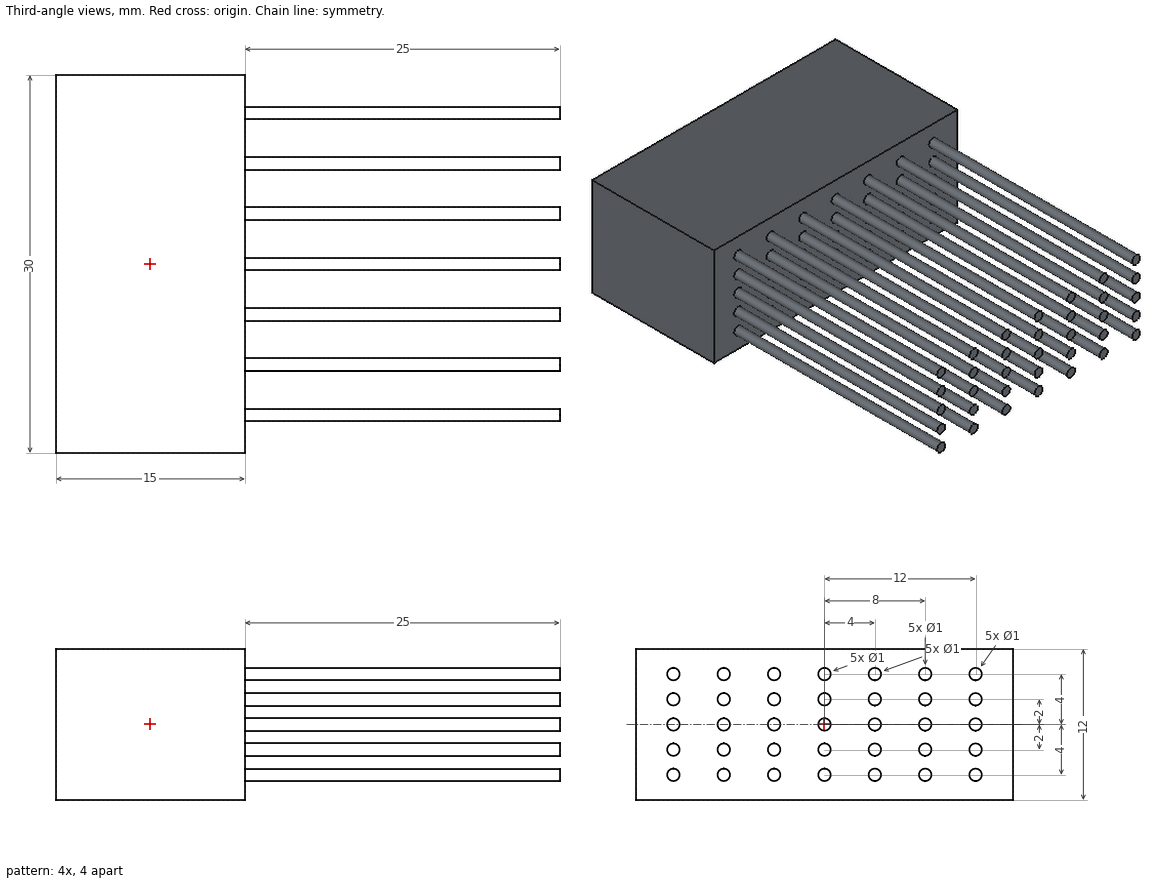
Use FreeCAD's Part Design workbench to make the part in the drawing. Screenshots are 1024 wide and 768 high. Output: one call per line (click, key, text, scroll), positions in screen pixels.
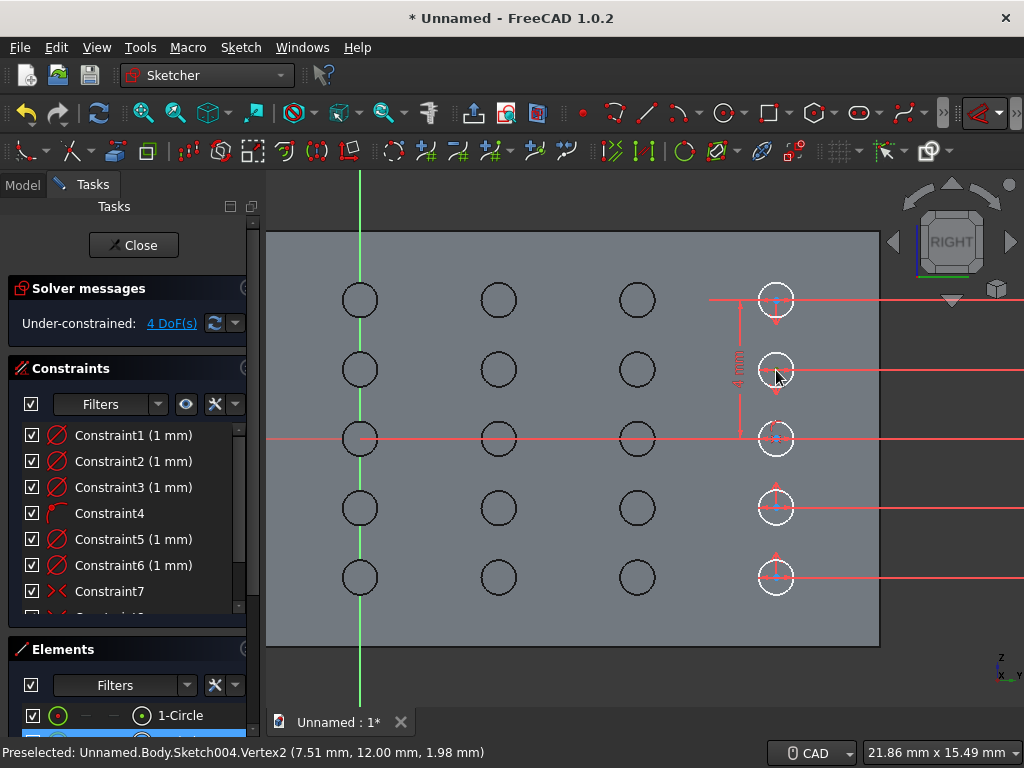
key(i)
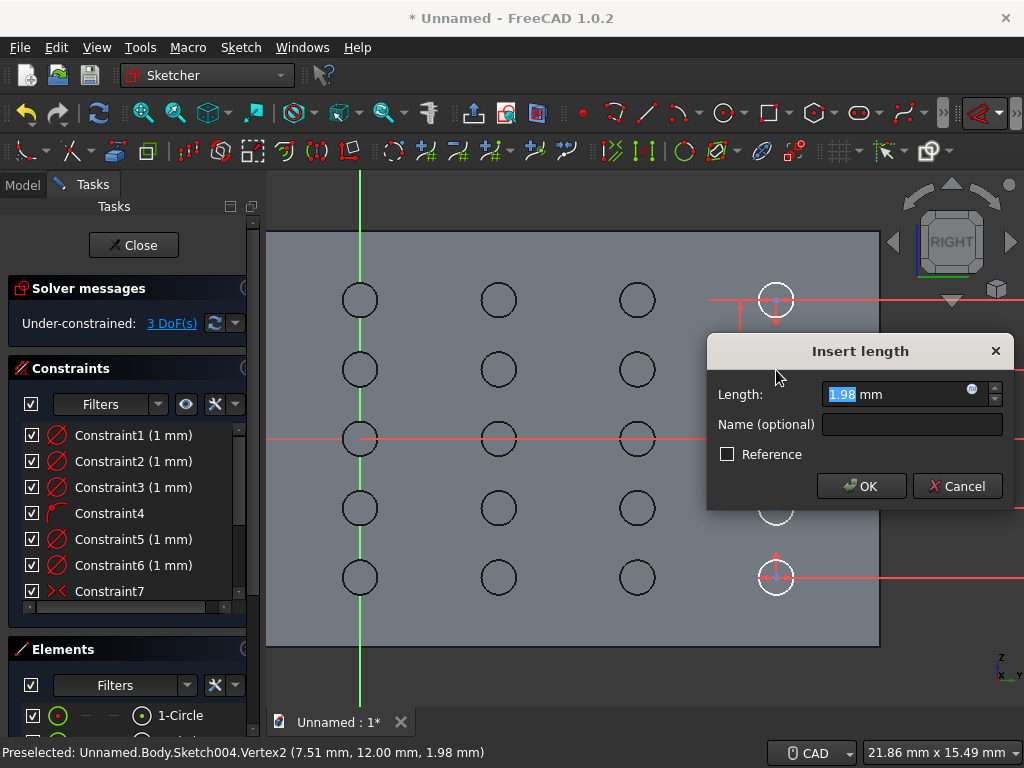
text(2)
key(Return)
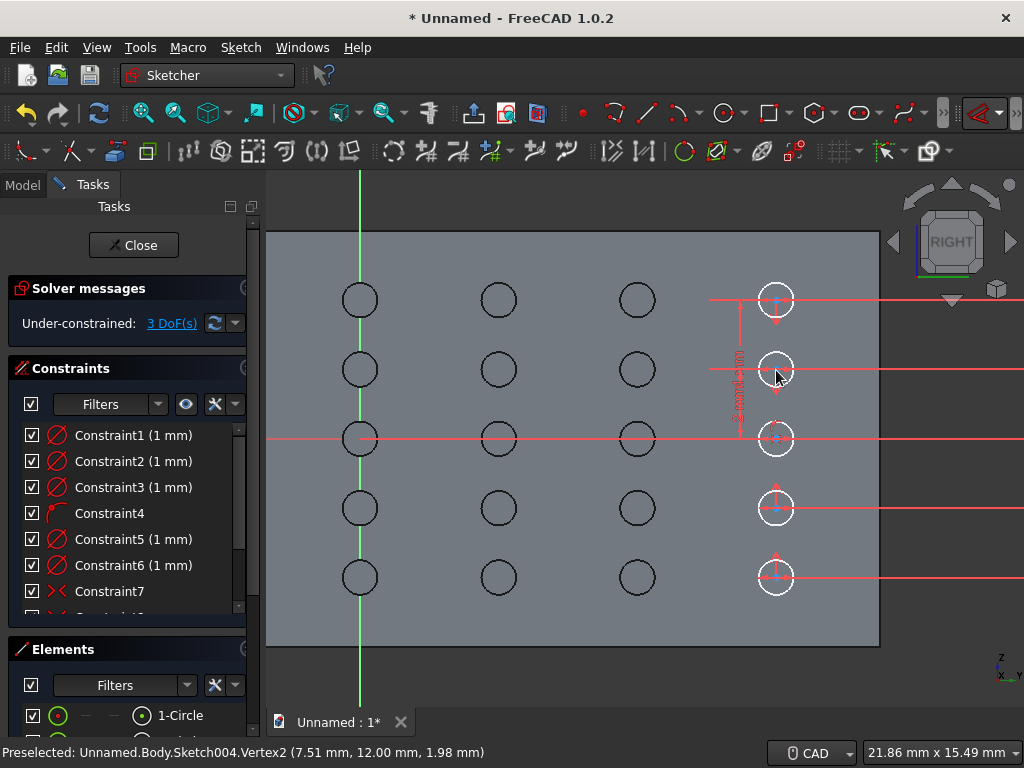
click(776, 300)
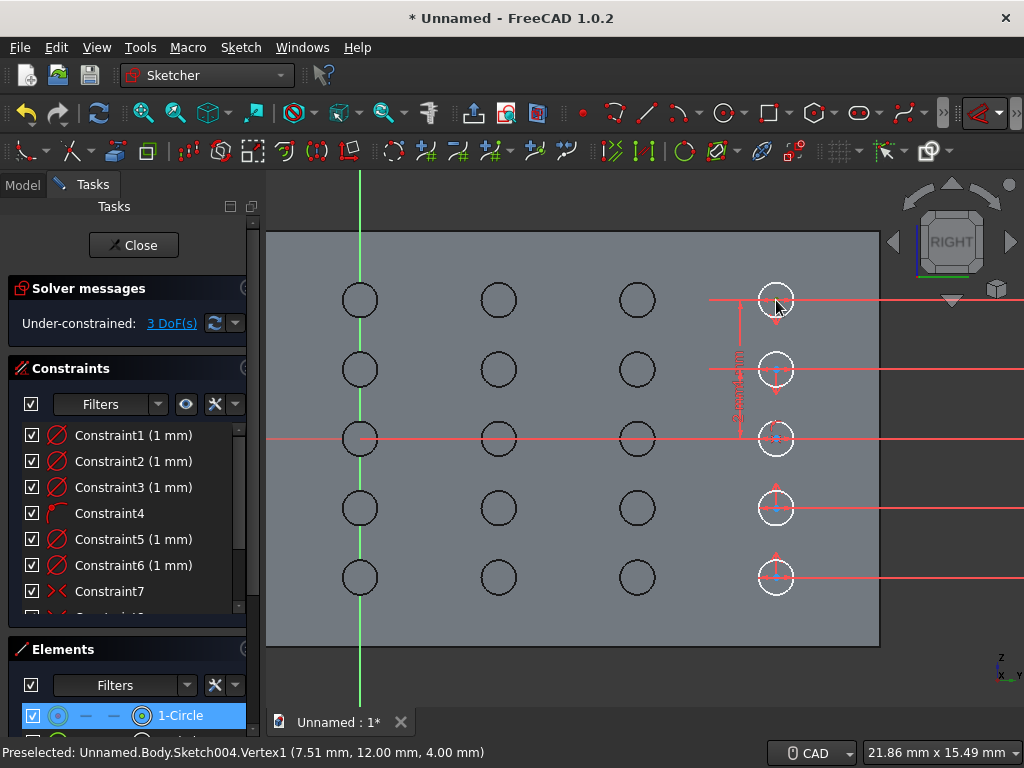
click(1002, 114)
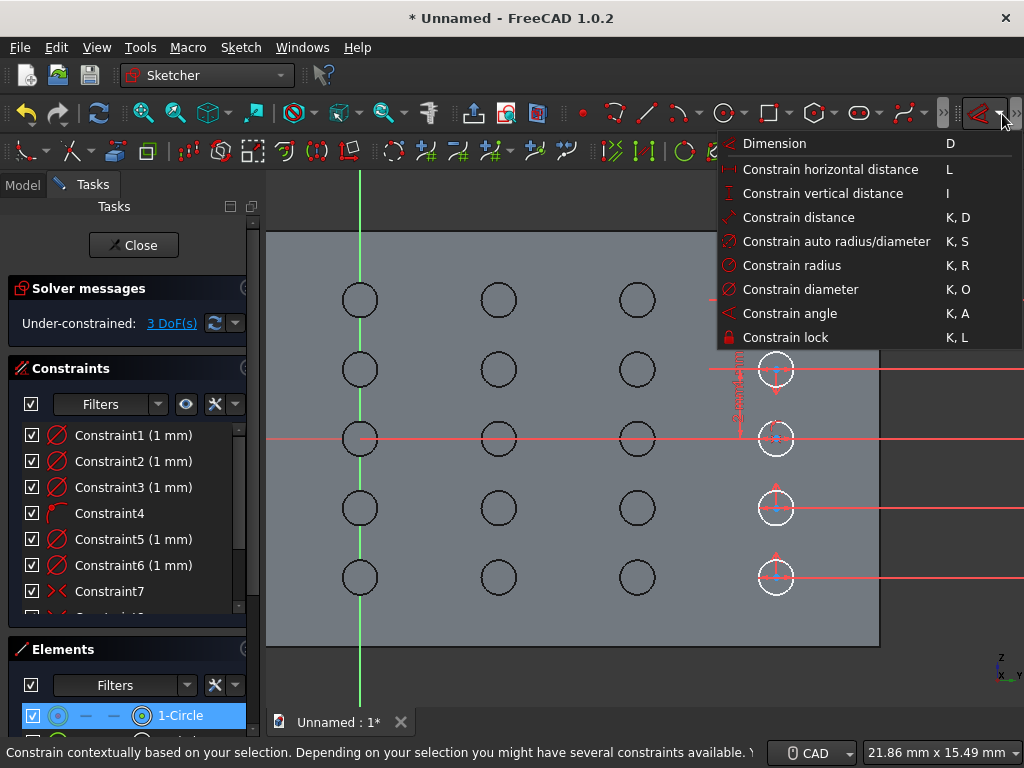
click(870, 169)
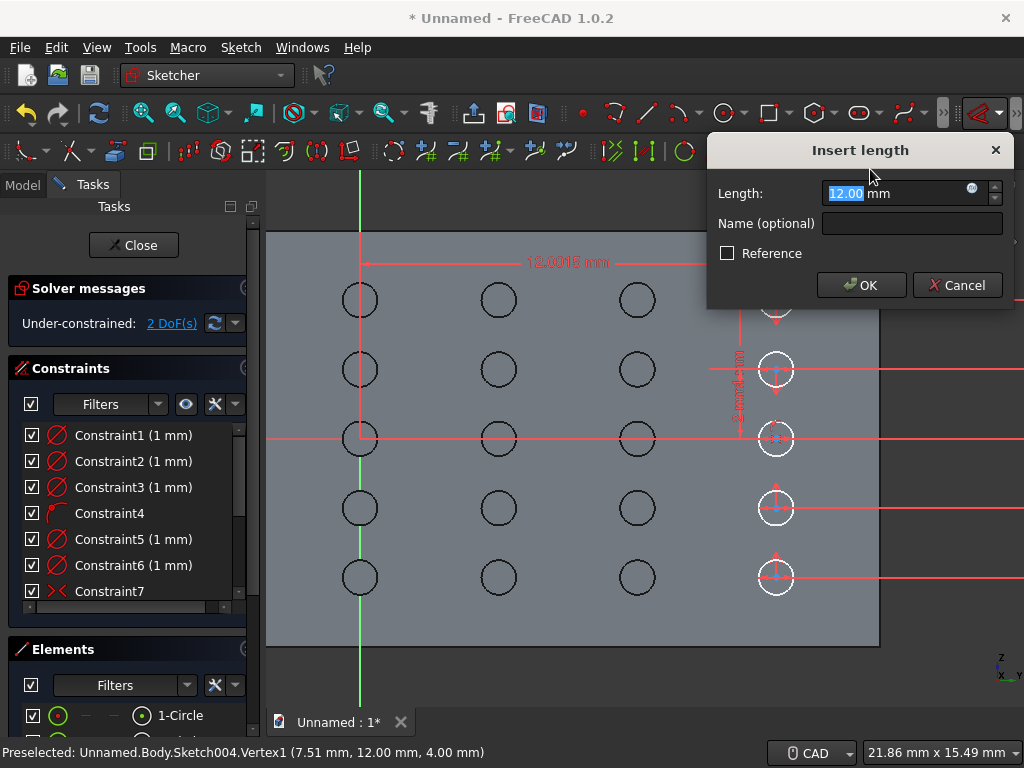
text(12)
key(Return)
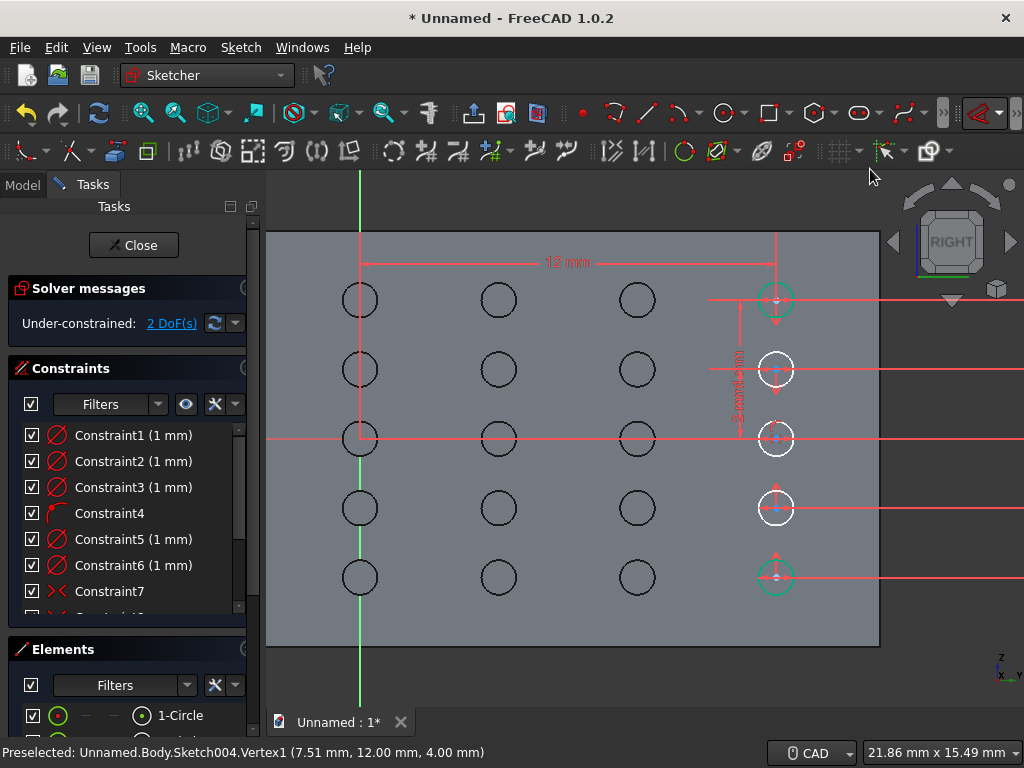
click(776, 369)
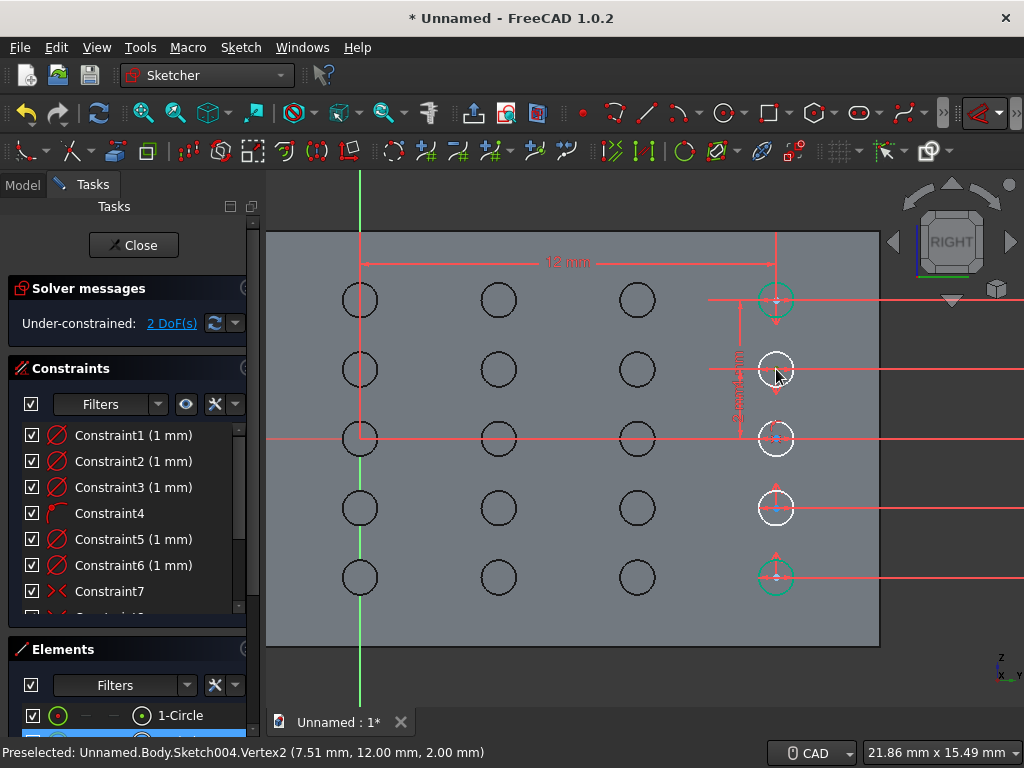
key(l)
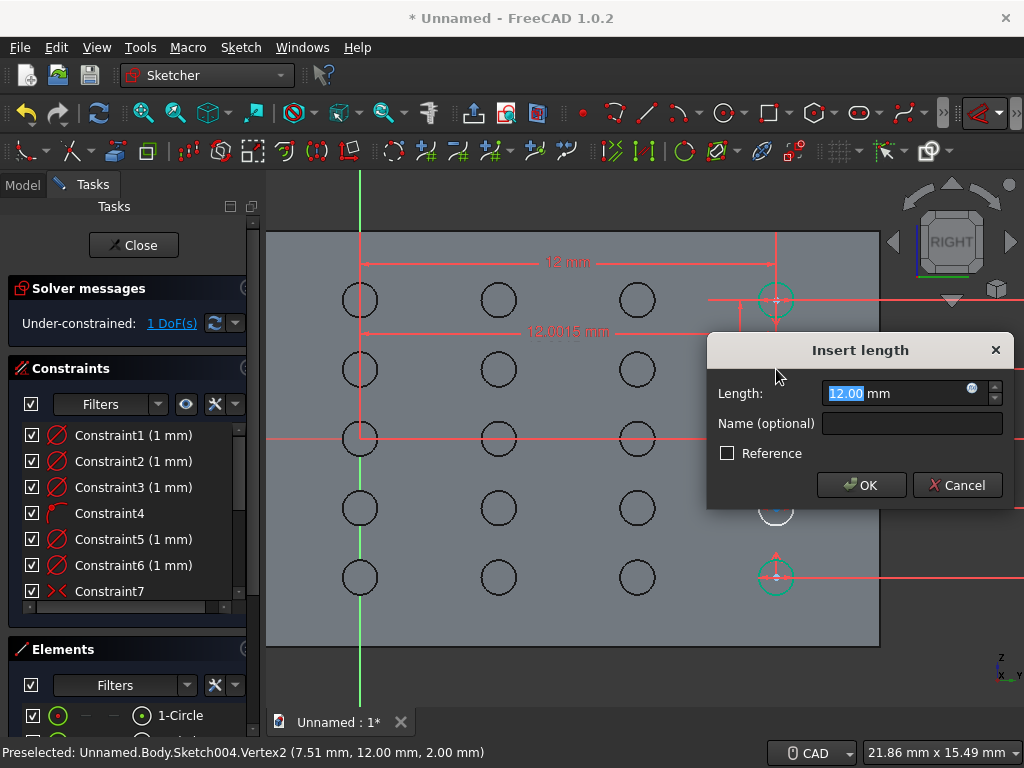
text(12)
key(Return)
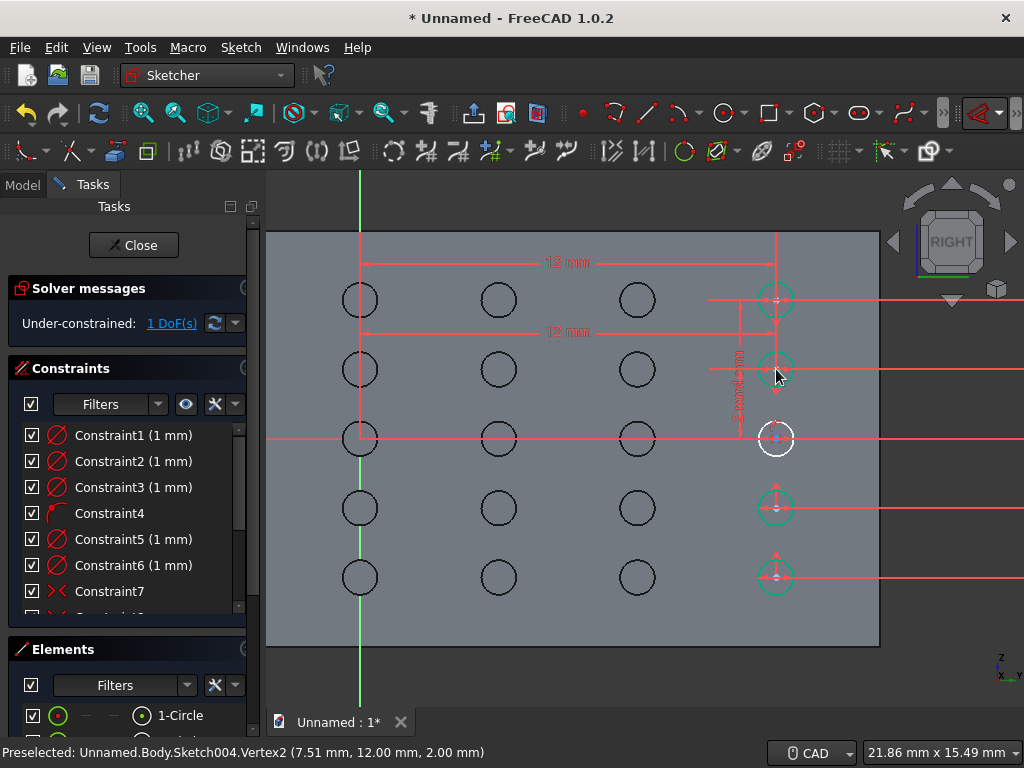
click(776, 439)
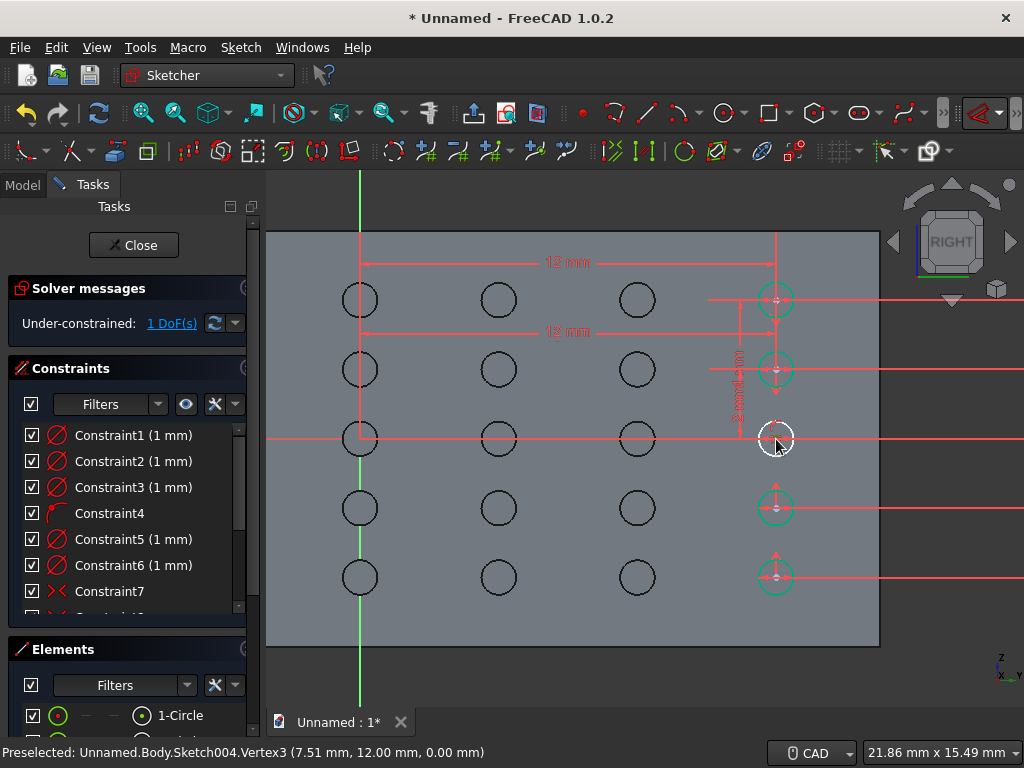
key(l)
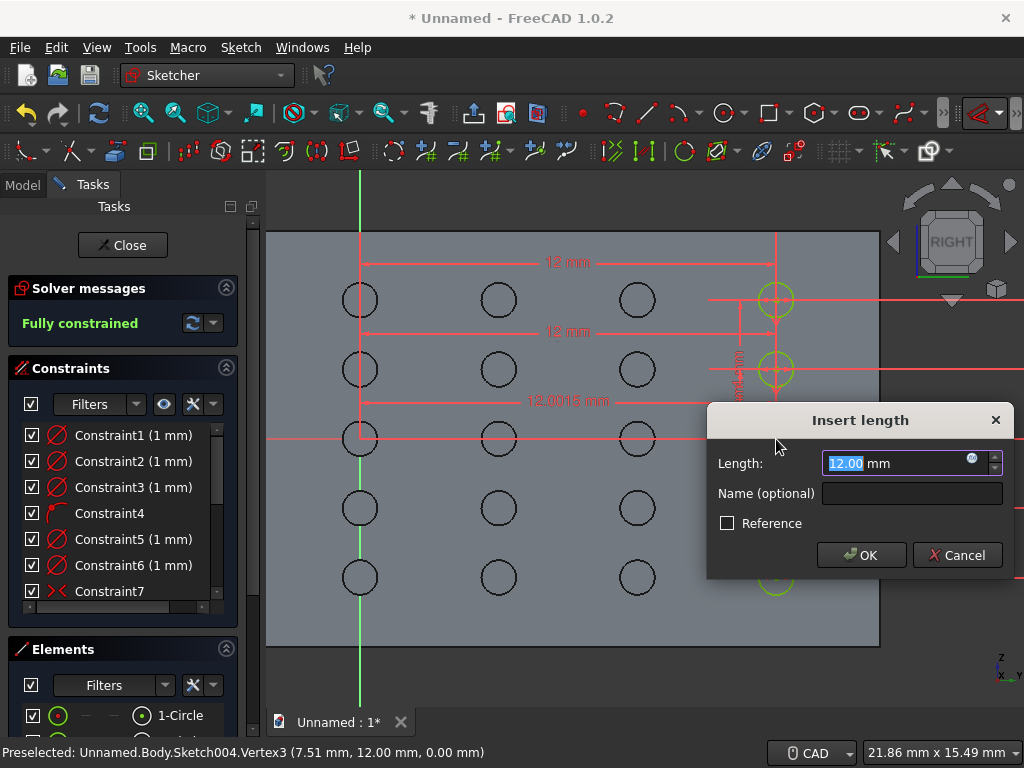
text(12)
key(Return)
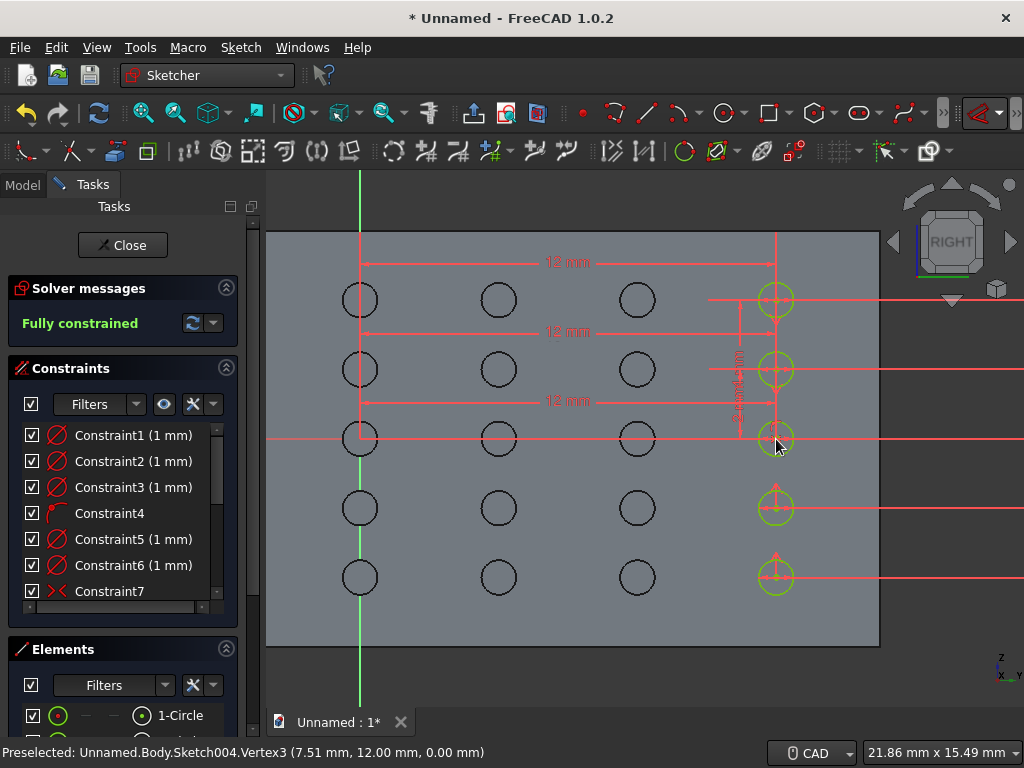
click(123, 245)